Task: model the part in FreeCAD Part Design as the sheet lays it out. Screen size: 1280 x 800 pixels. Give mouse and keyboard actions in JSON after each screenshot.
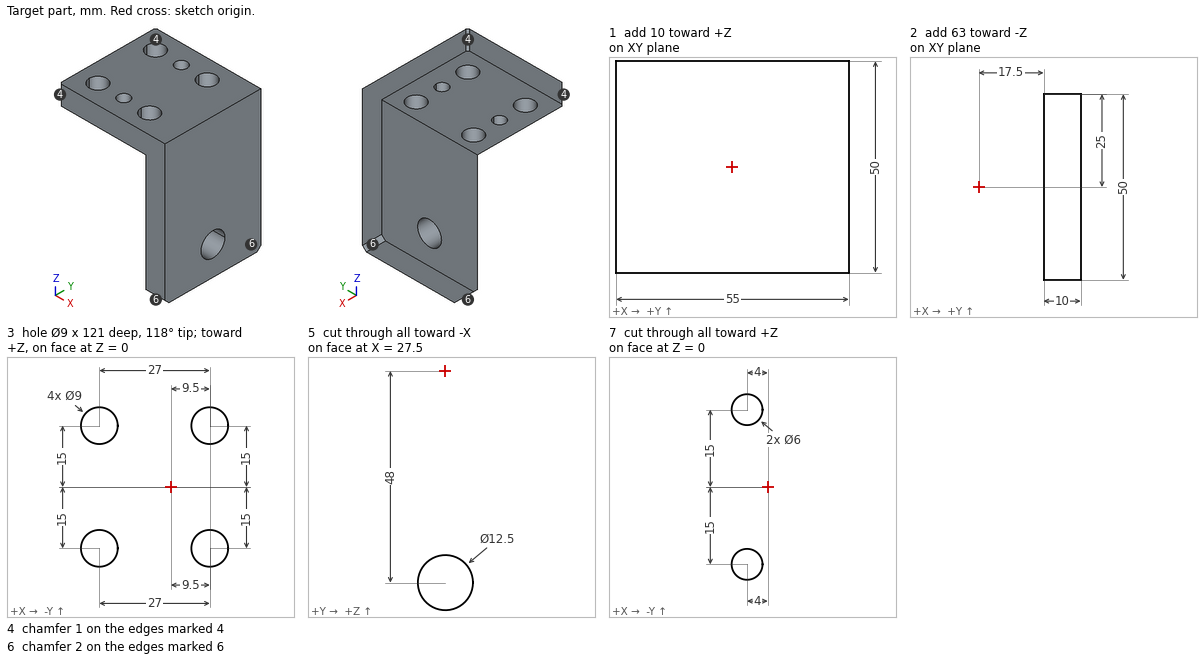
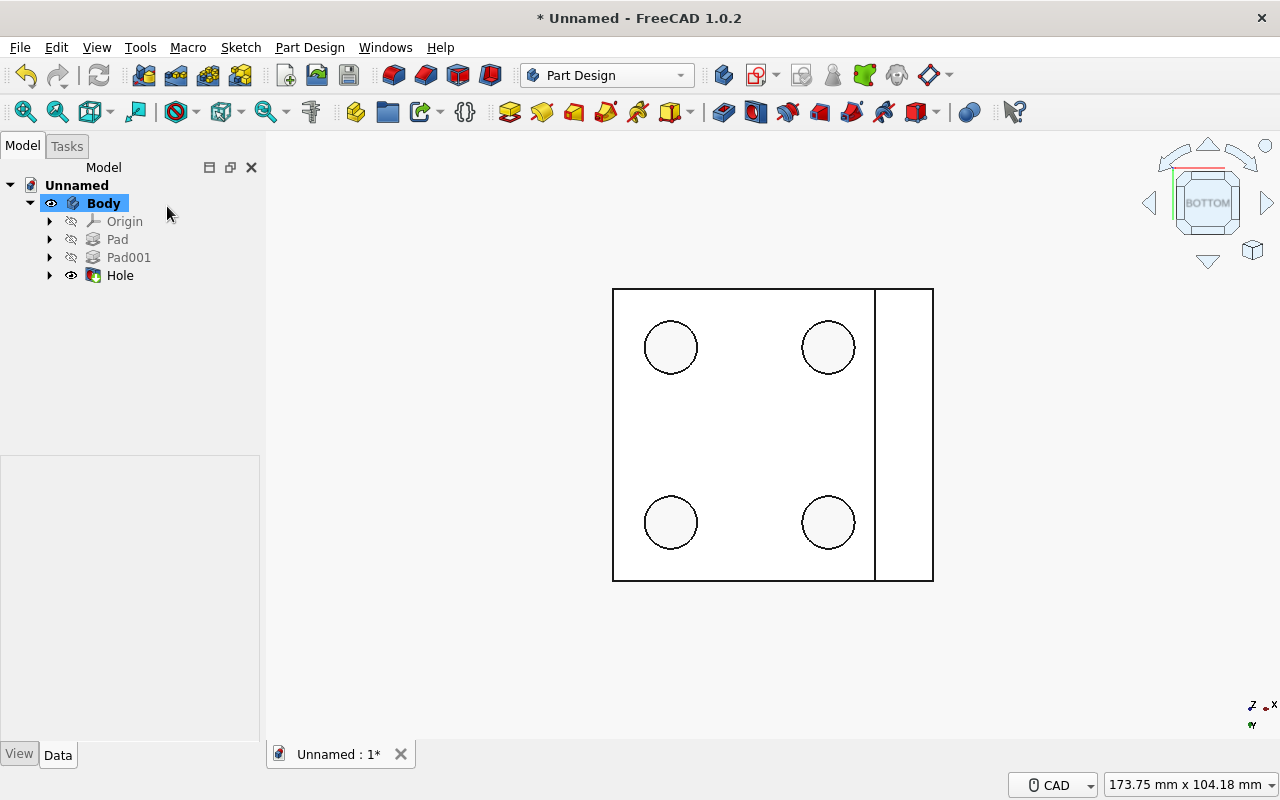
{"action": "key", "text": "0"}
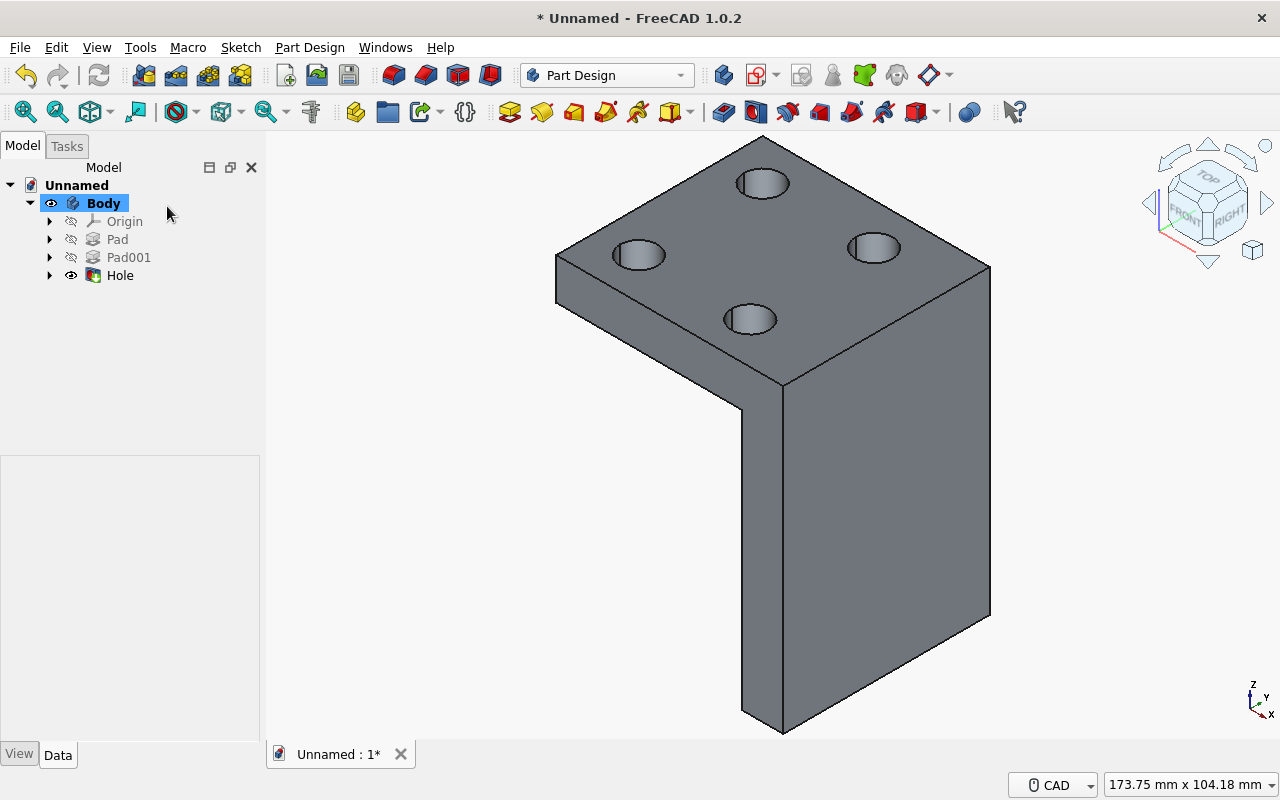
{"action": "key", "text": "2"}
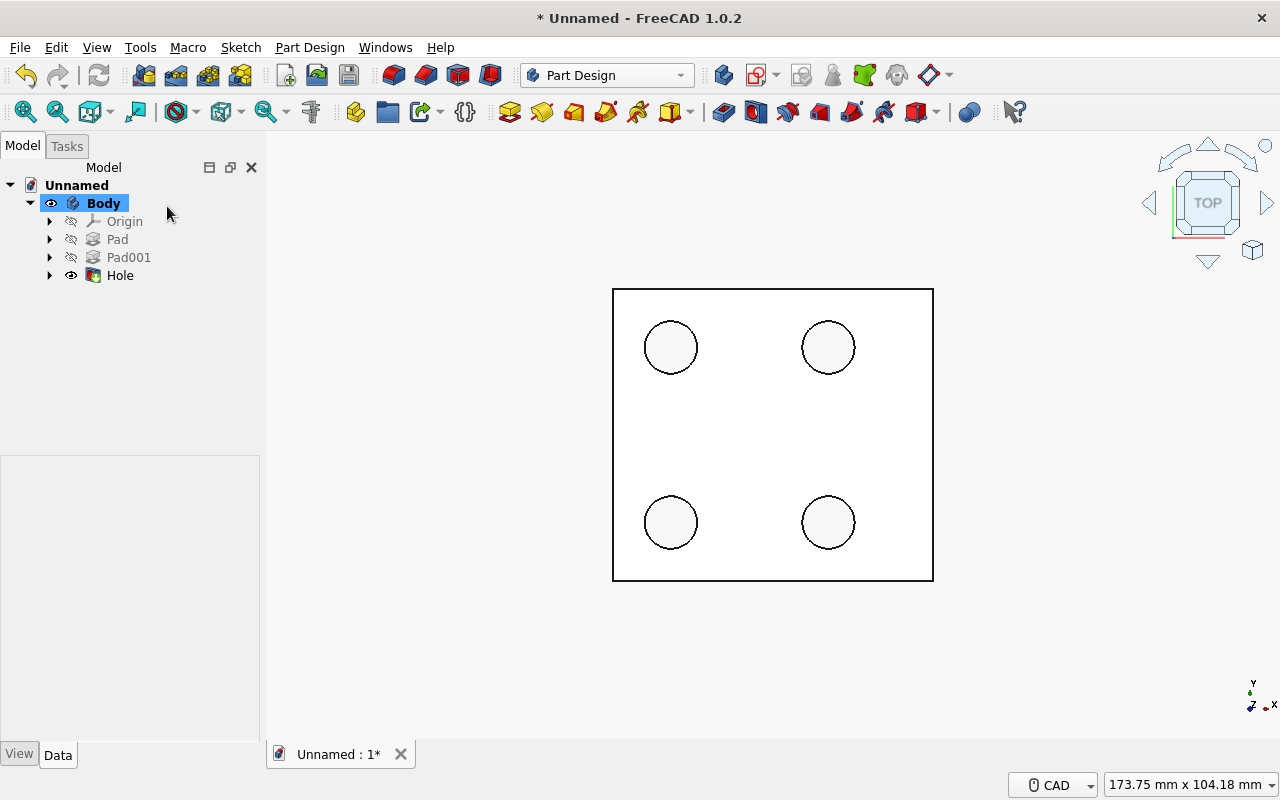
{"action": "key", "text": "1"}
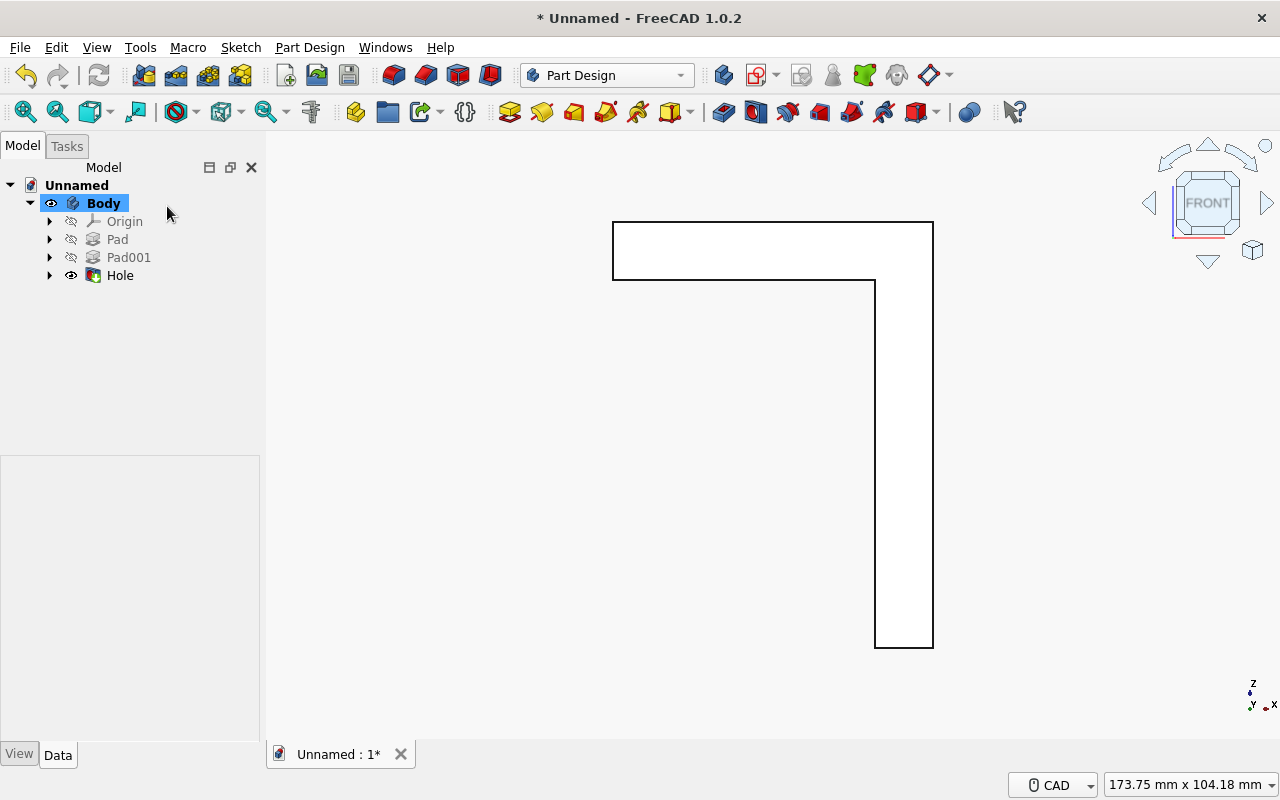
{"action": "left_click", "coordinate": [613, 250]}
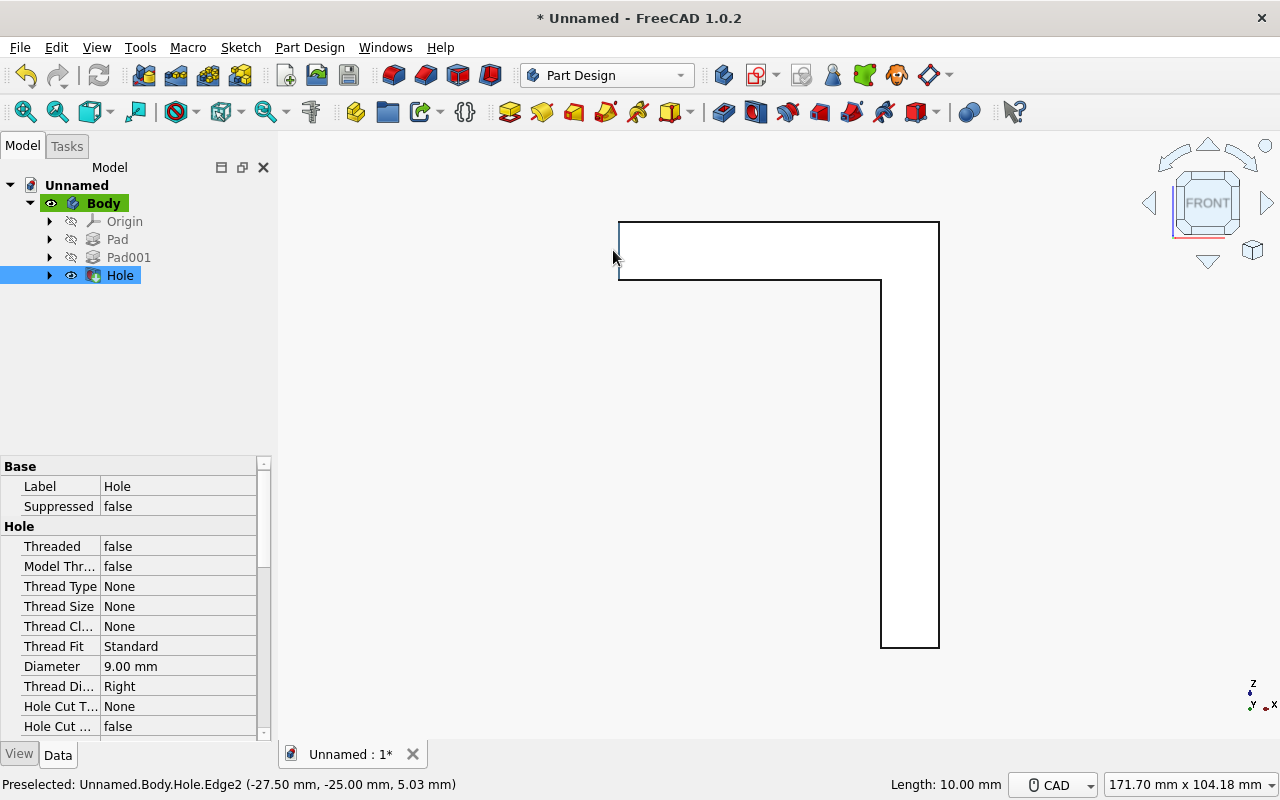
{"action": "key", "text": "3"}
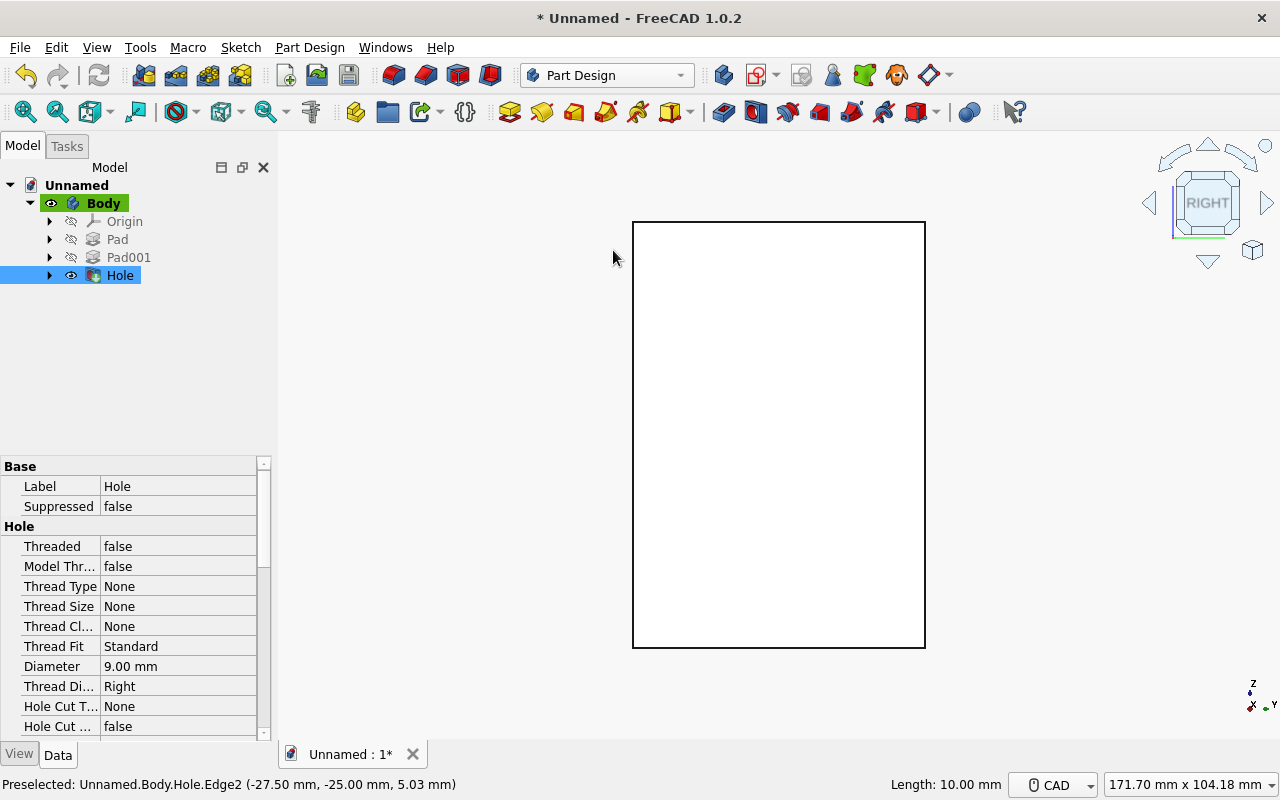
{"action": "key", "text": "5"}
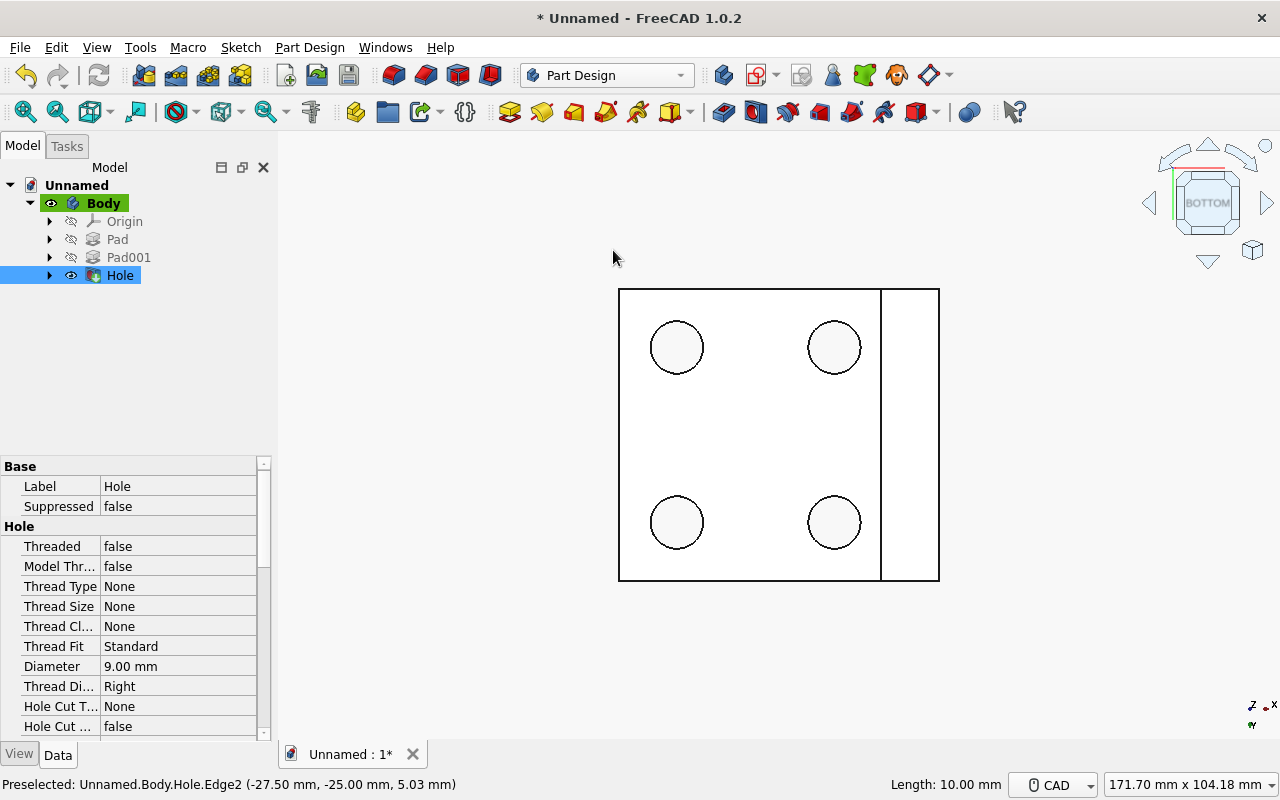
{"action": "key", "text": "4"}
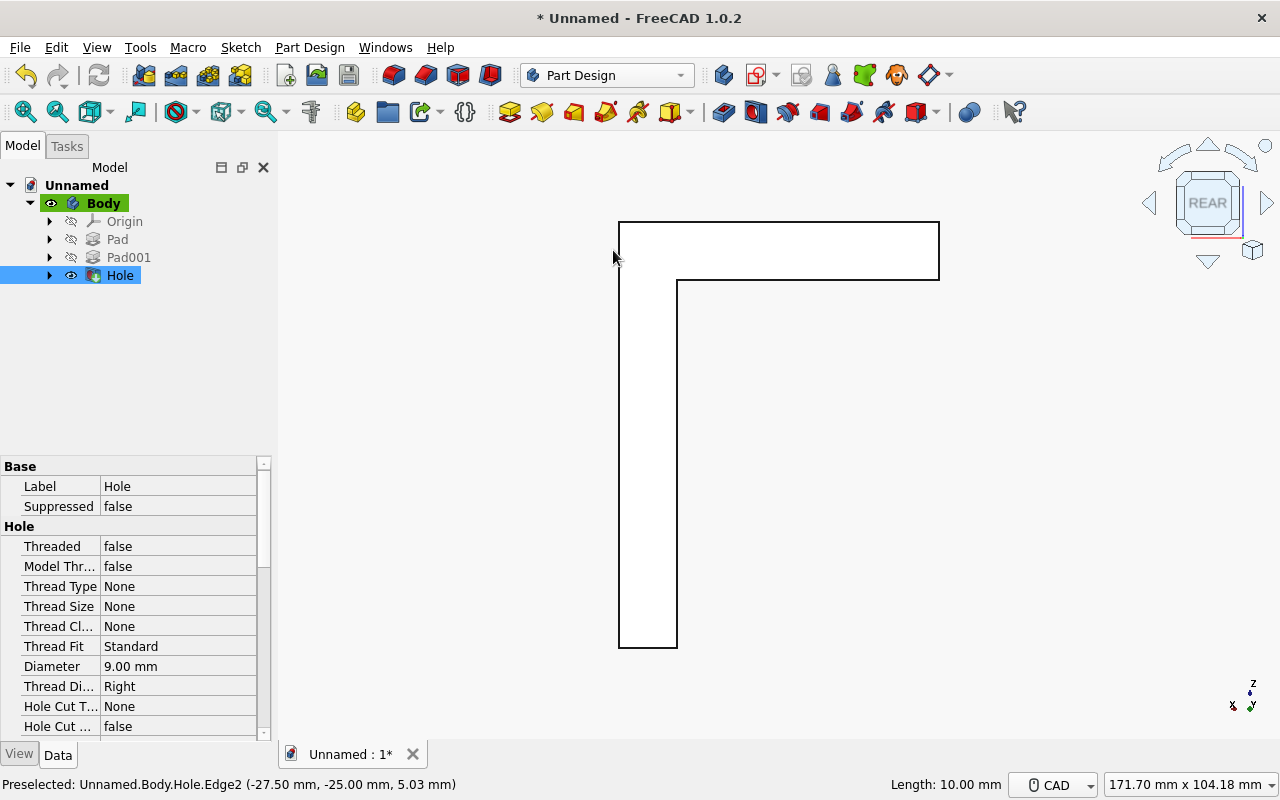
{"action": "left_click", "coordinate": [939, 250], "text": "ctrl"}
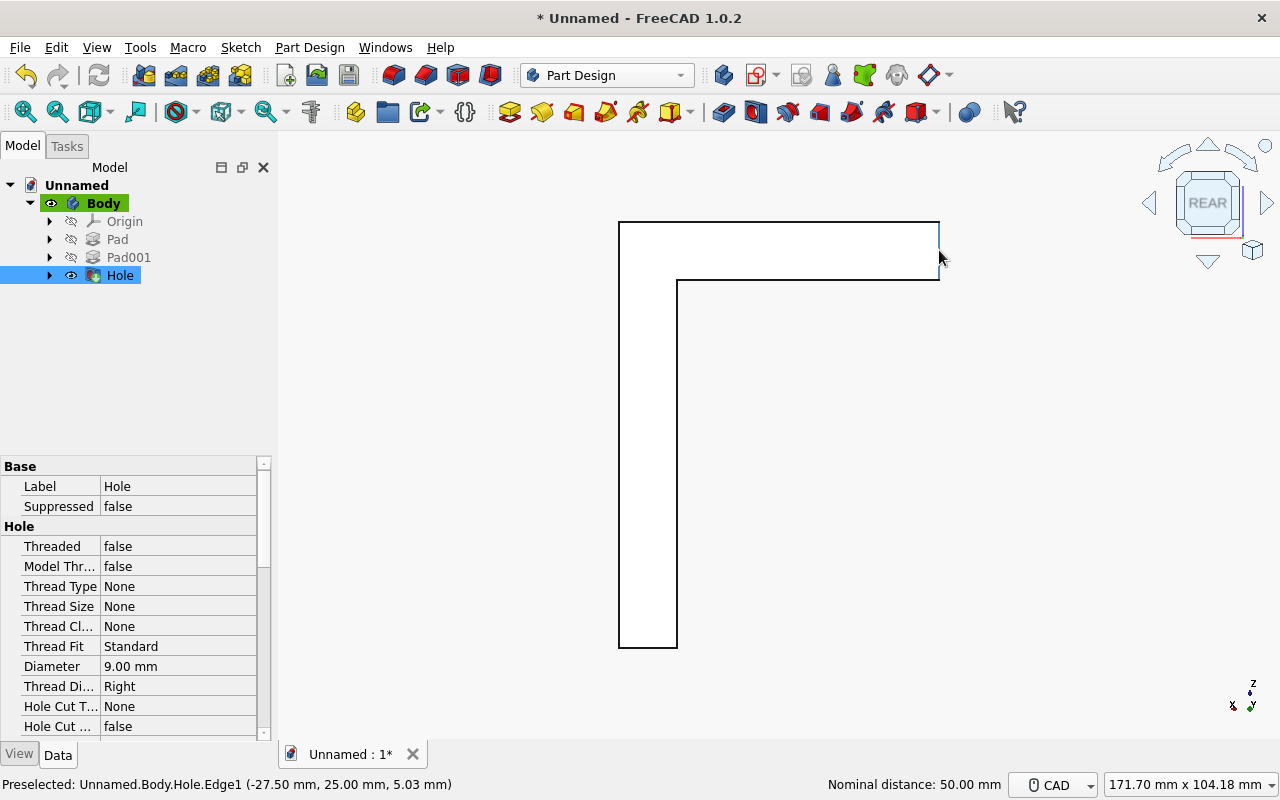
{"action": "left_click", "coordinate": [426, 76]}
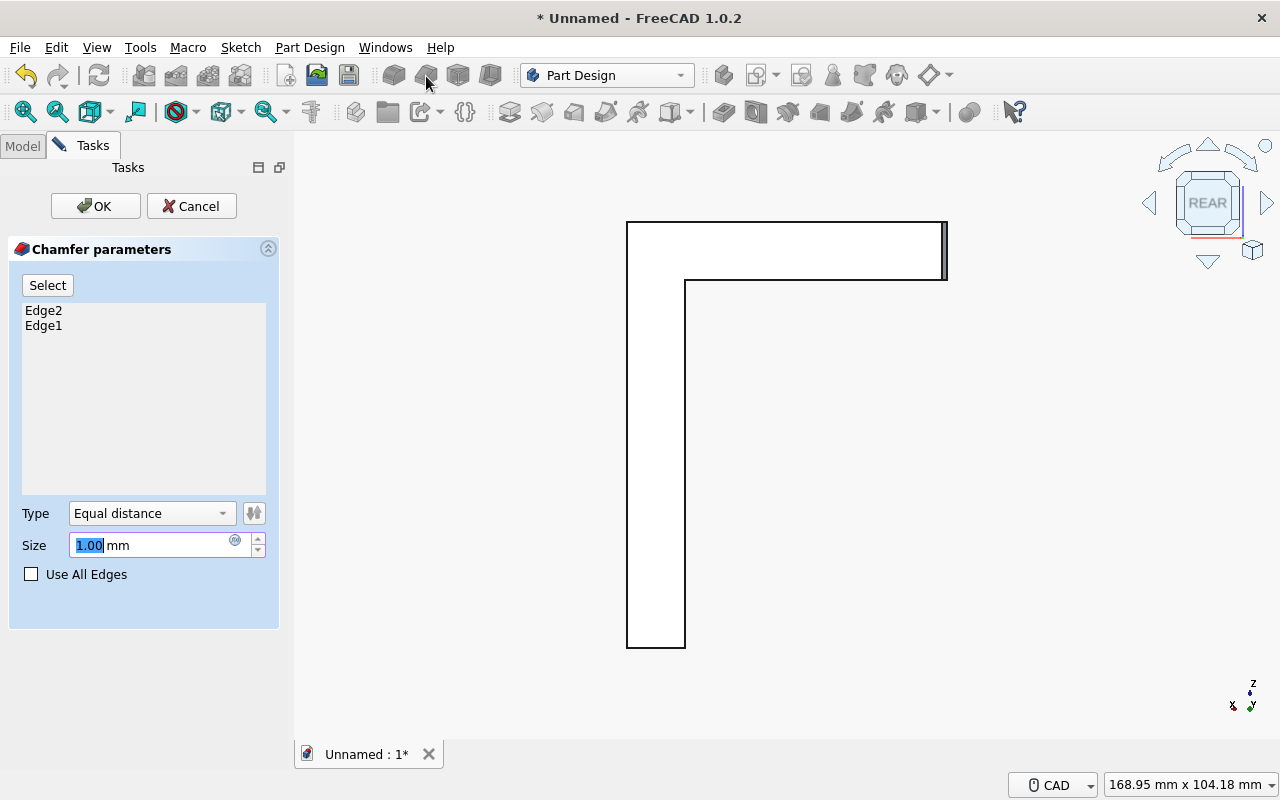
{"action": "type", "text": "1"}
{"action": "key", "text": "Tab"}